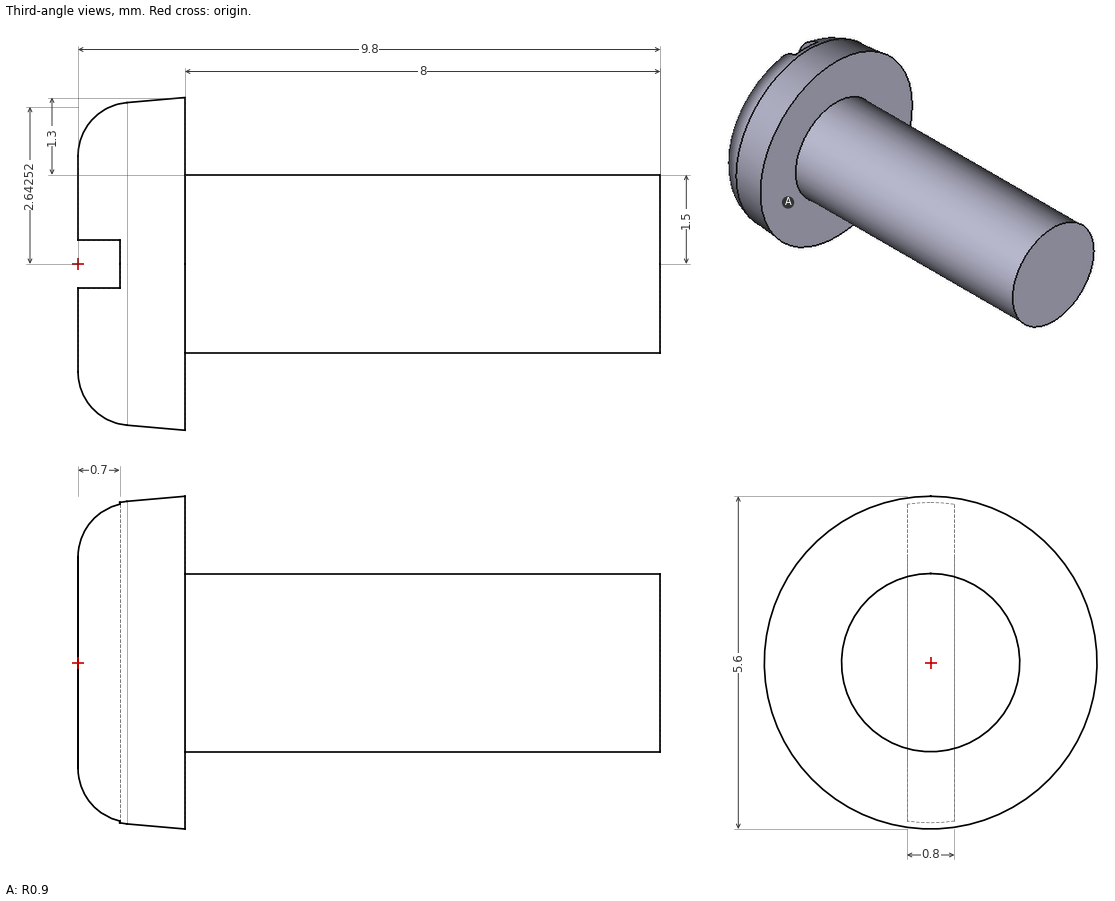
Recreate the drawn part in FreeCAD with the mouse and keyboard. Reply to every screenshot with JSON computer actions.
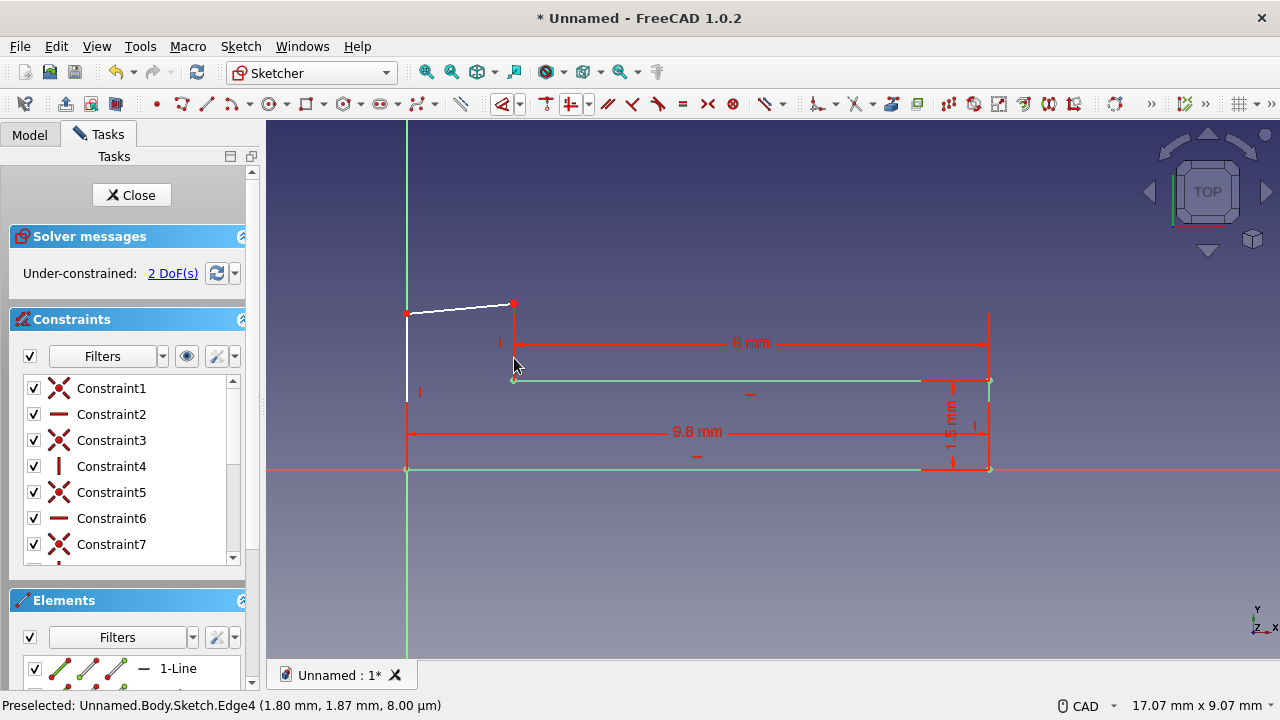
{"action": "left_click", "coordinate": [520, 104]}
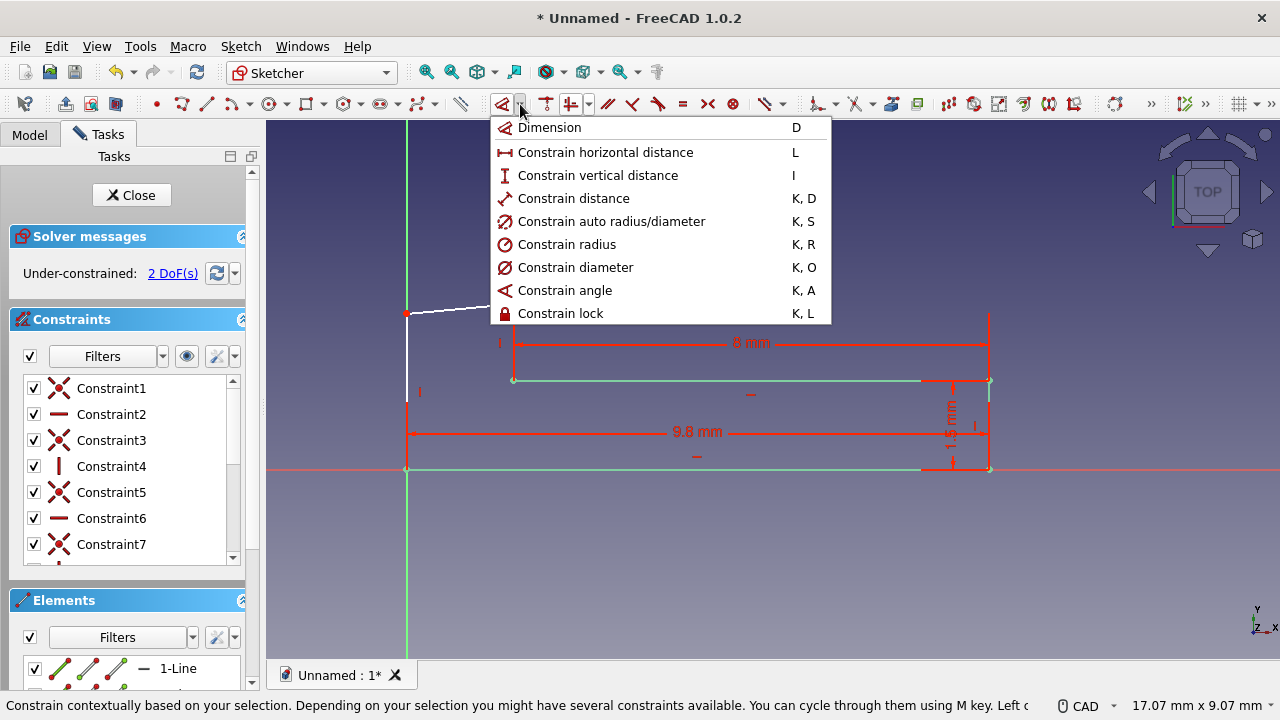
{"action": "left_click", "coordinate": [661, 176]}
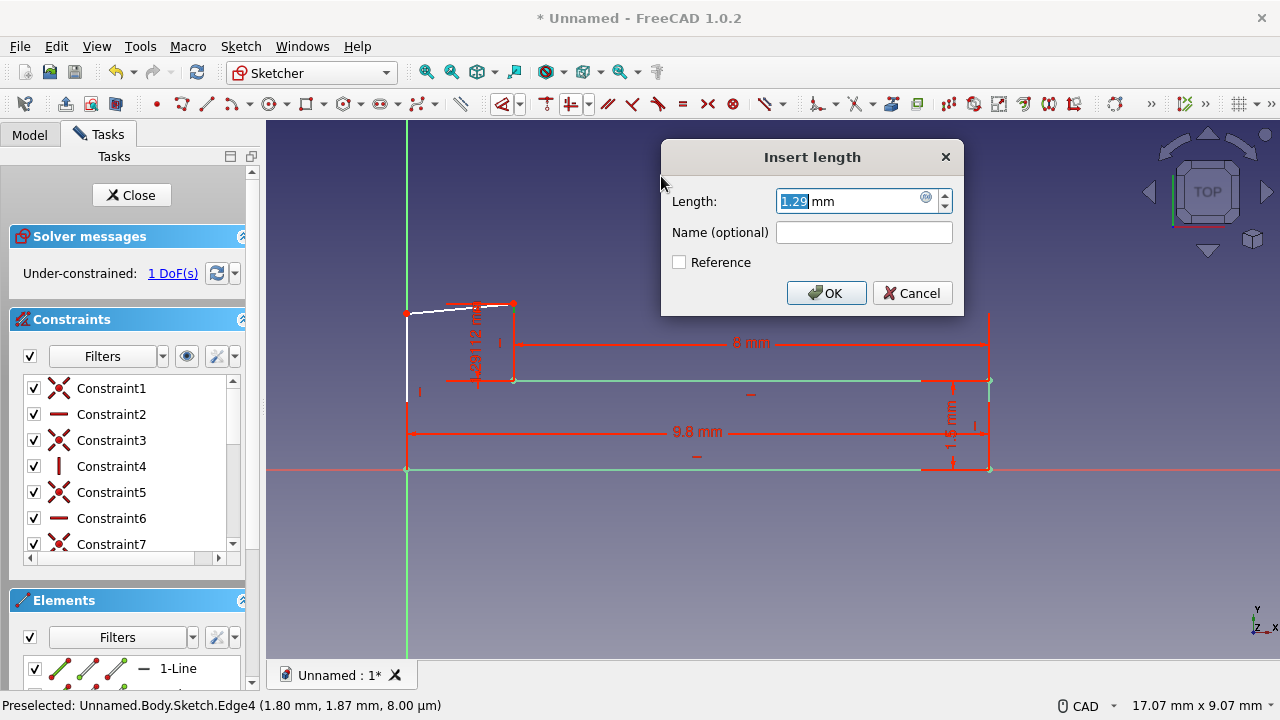
{"action": "type", "text": "1.3"}
{"action": "key", "text": "Return"}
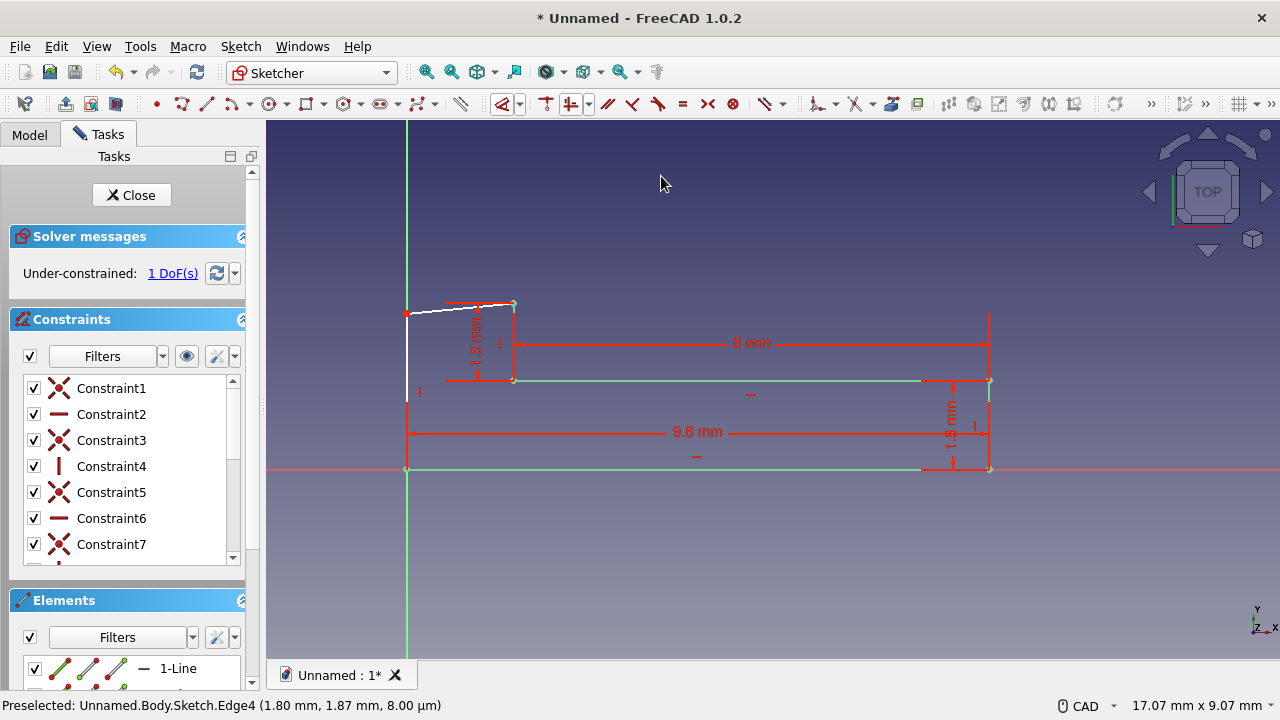
{"action": "left_click", "coordinate": [407, 361]}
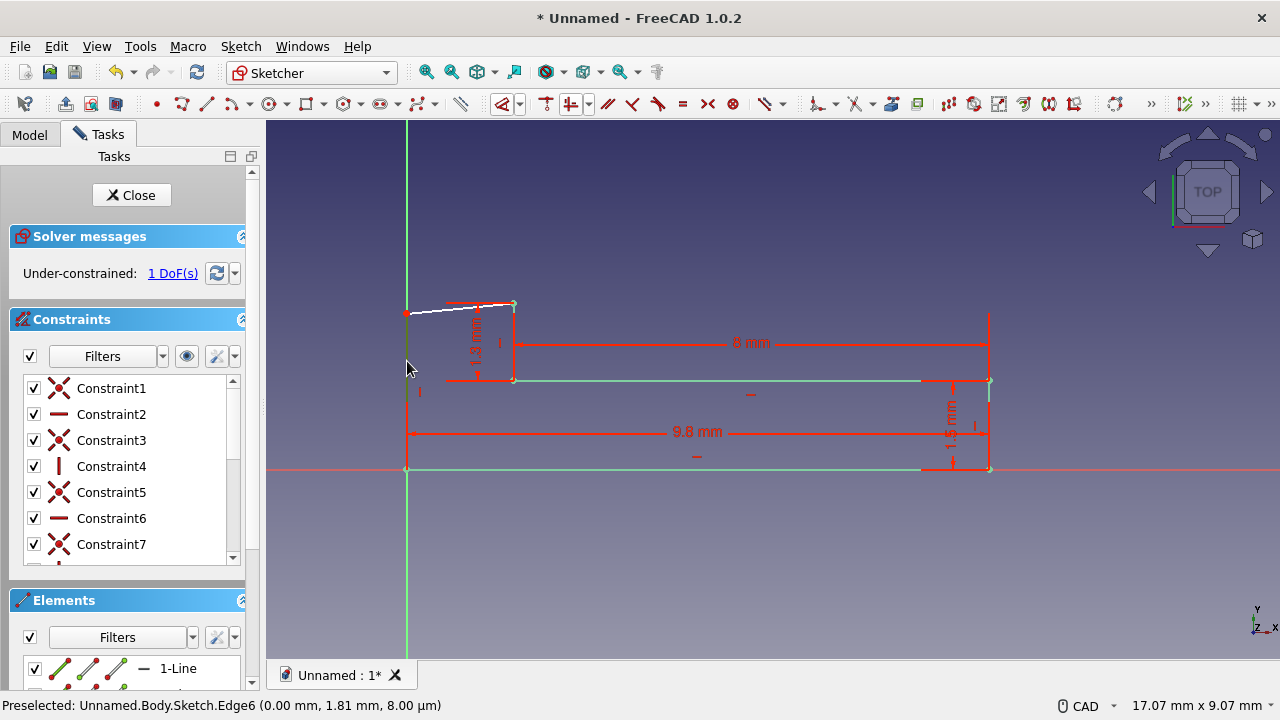
{"action": "key", "text": "i"}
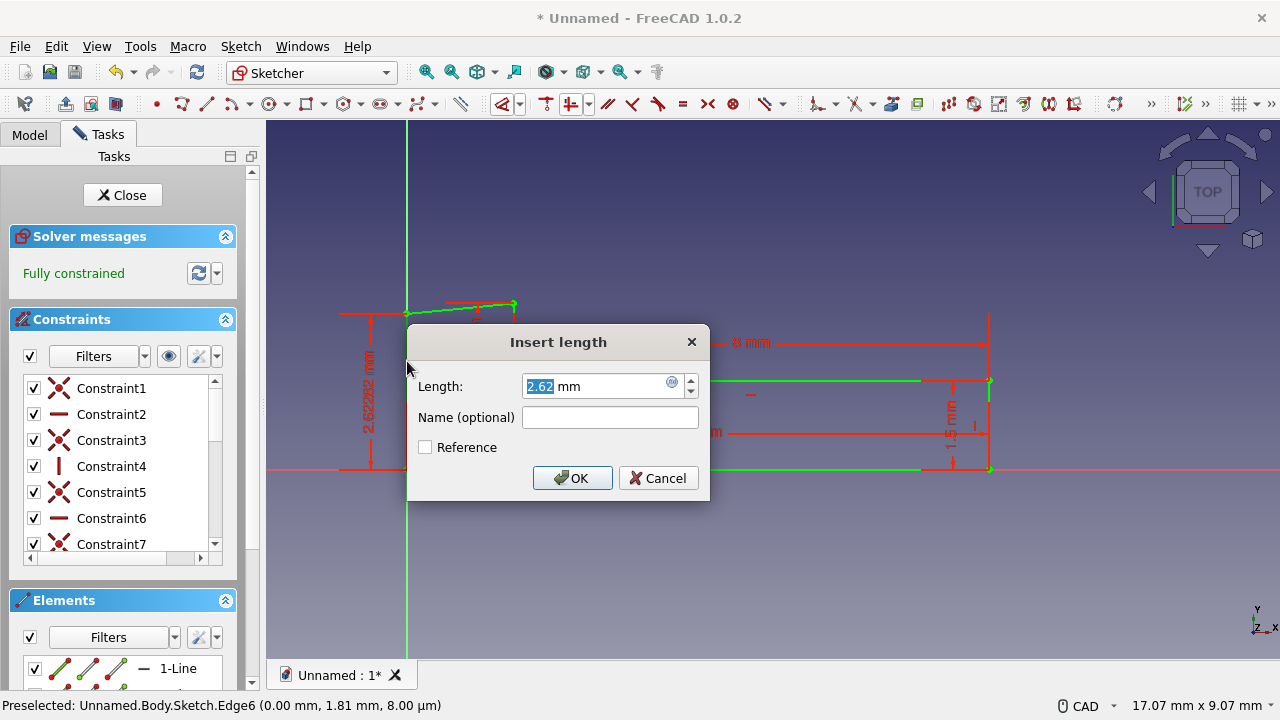
{"action": "type", "text": "2.64252"}
{"action": "key", "text": "Return"}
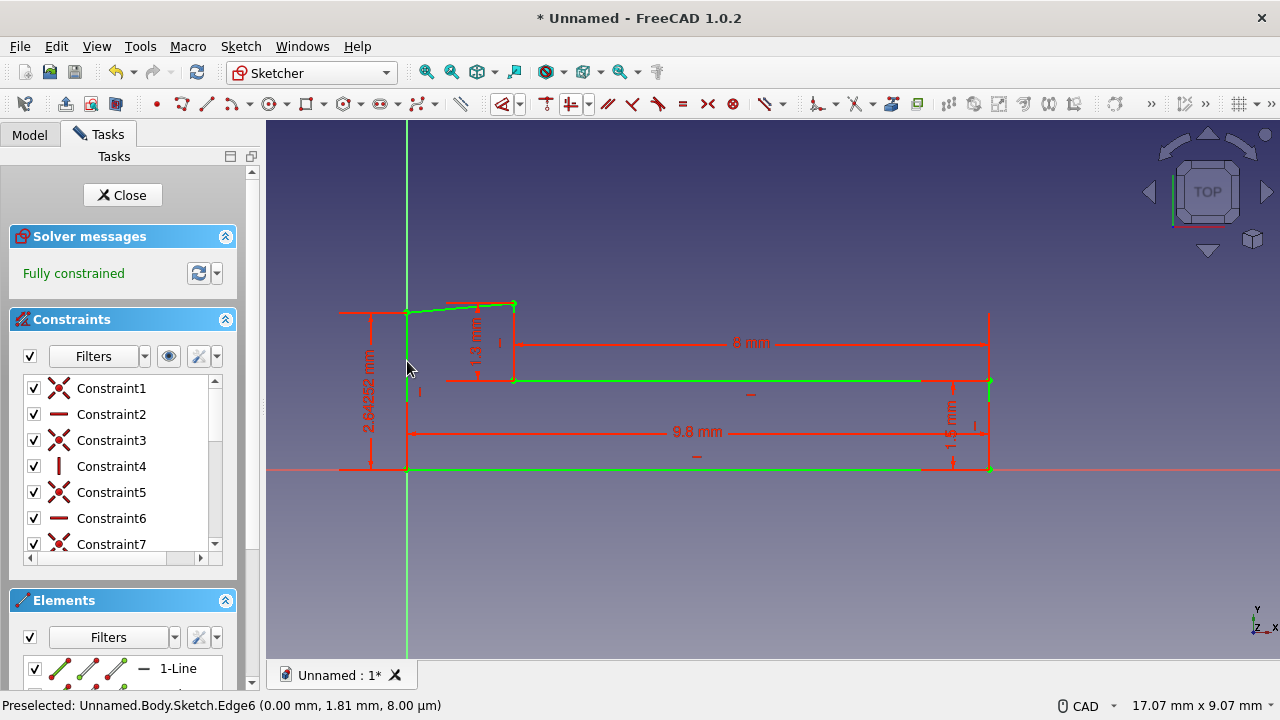
{"action": "left_click", "coordinate": [123, 195]}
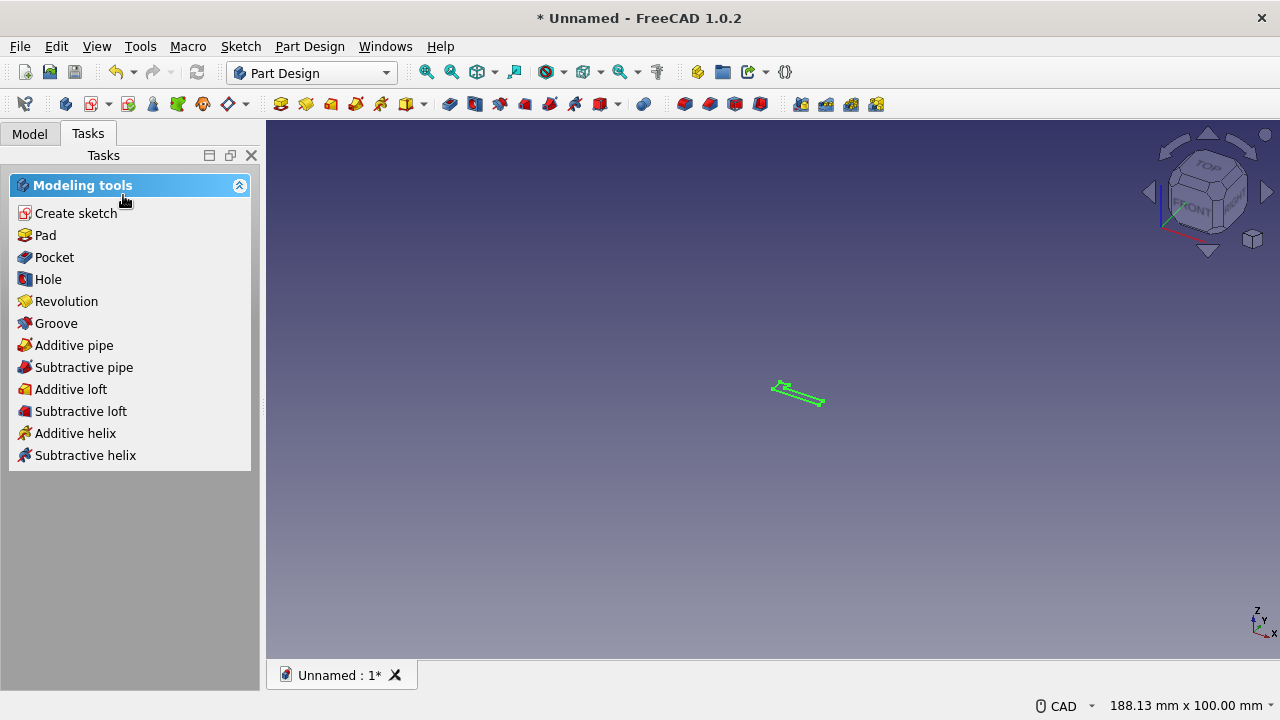
{"action": "left_click", "coordinate": [306, 104]}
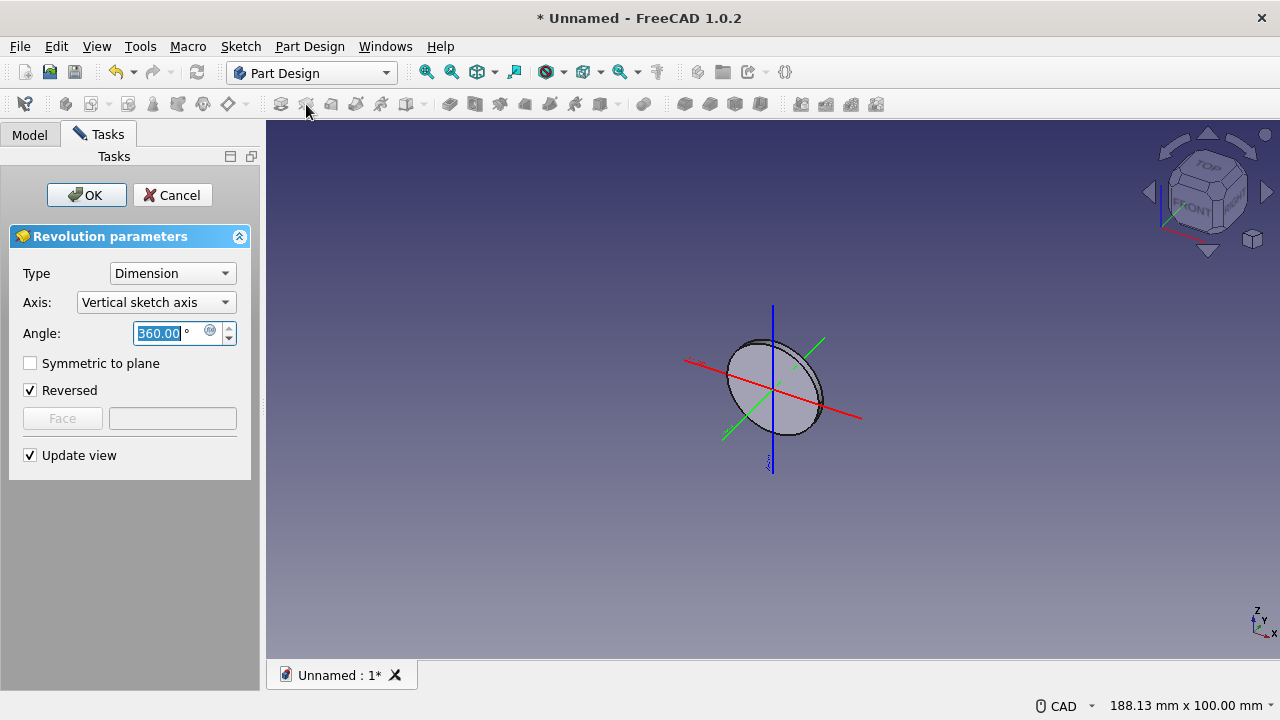
{"action": "left_click", "coordinate": [157, 302]}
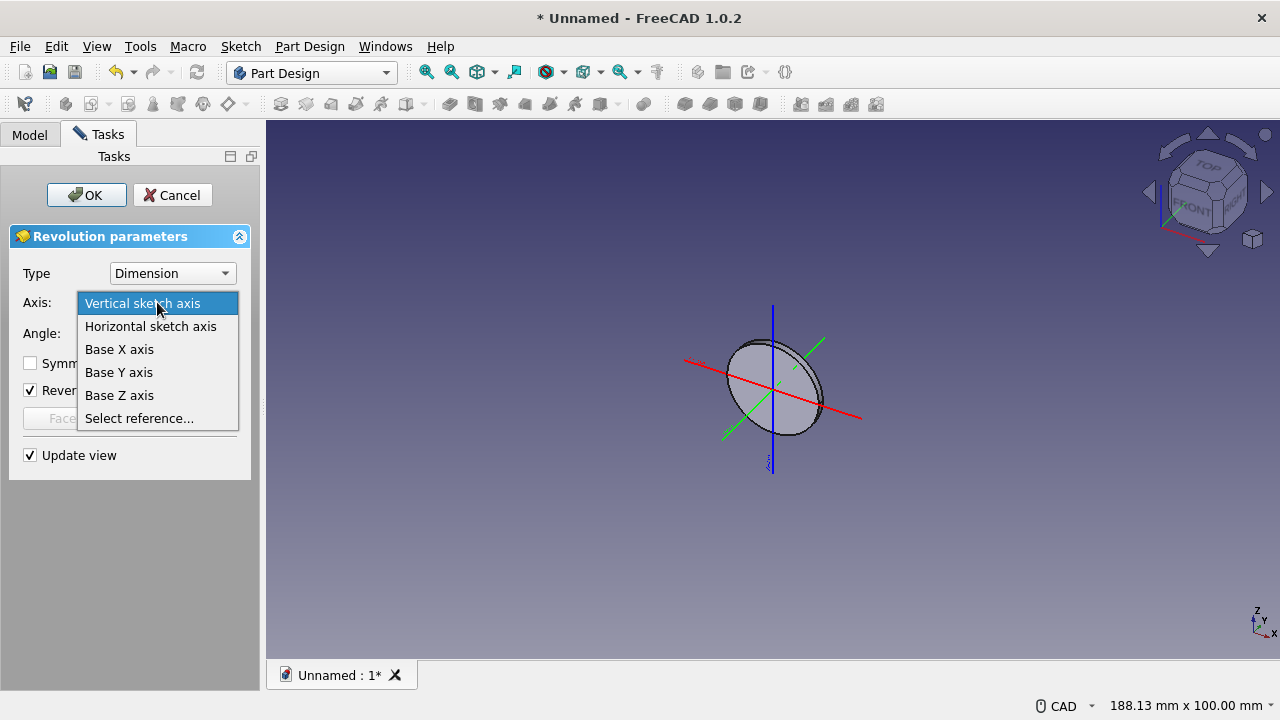
{"action": "left_click", "coordinate": [156, 326]}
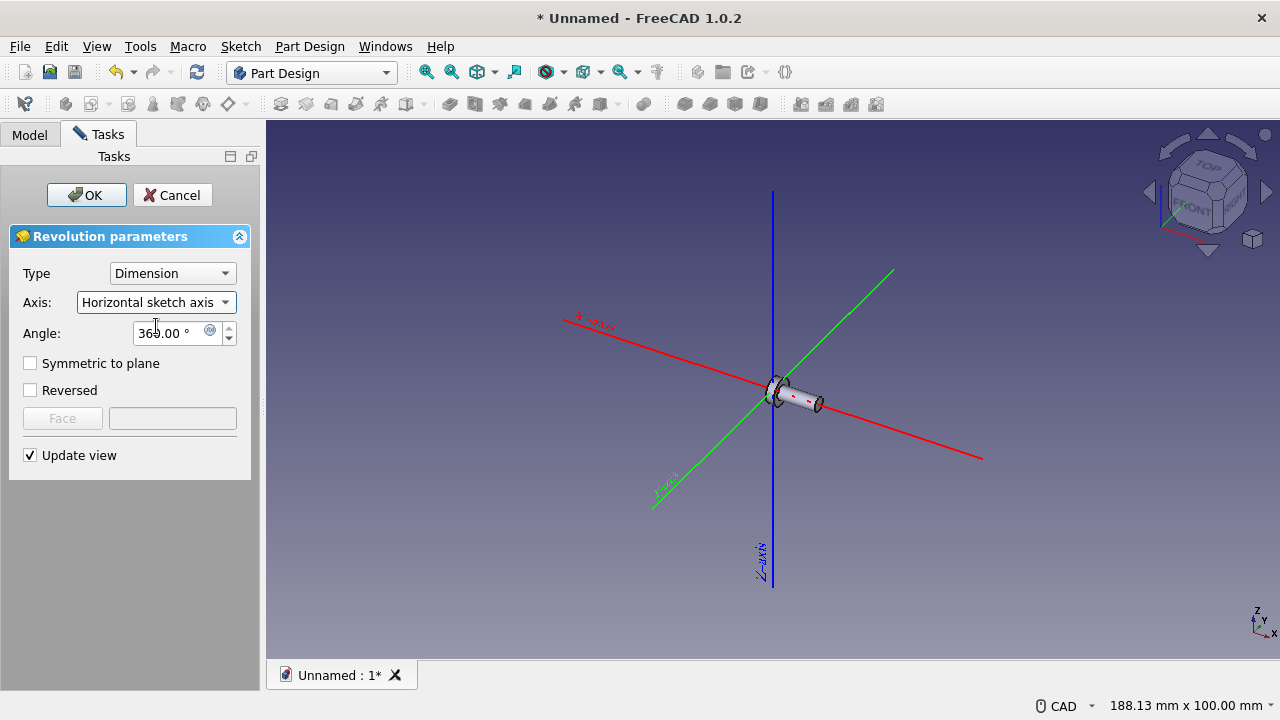
{"action": "left_click", "coordinate": [87, 195]}